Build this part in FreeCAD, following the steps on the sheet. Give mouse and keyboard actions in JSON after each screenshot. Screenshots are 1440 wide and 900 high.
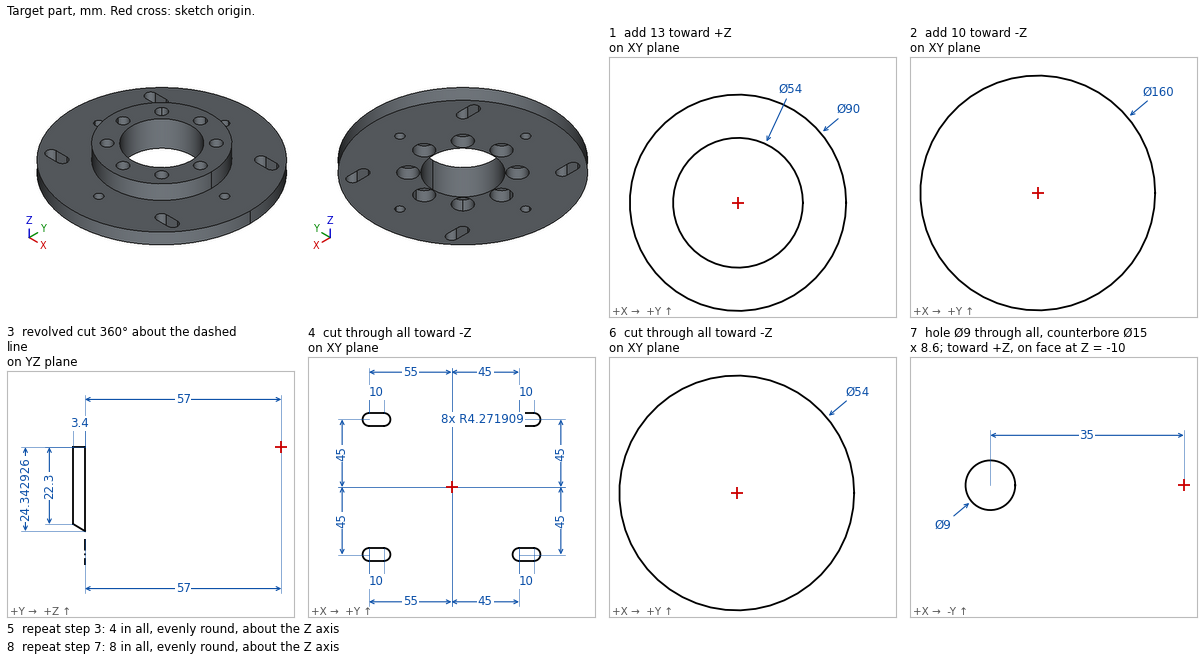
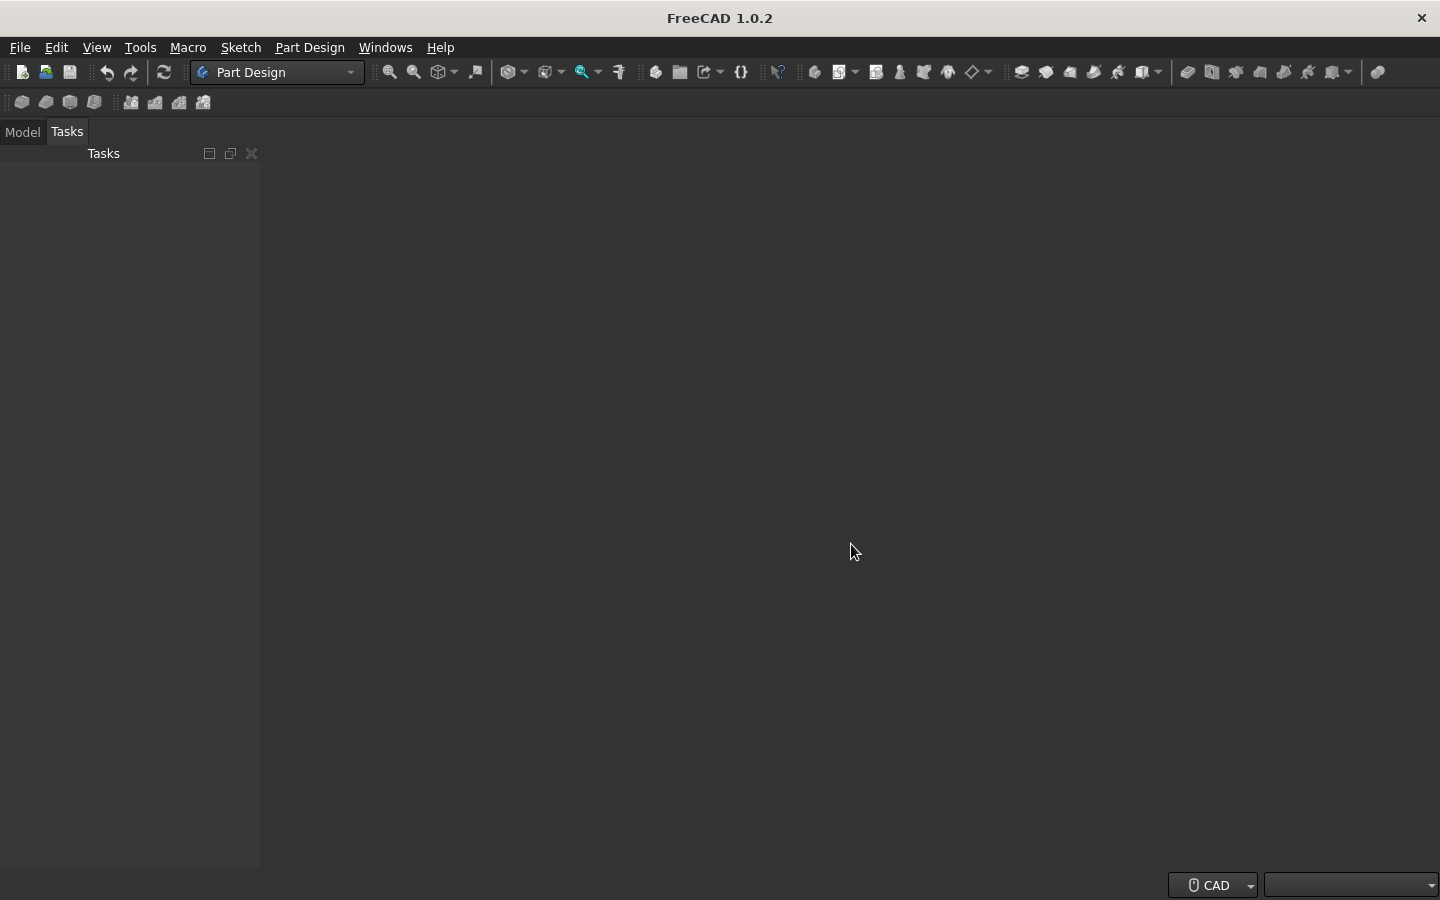
{"action": "key", "text": "ctrl+n"}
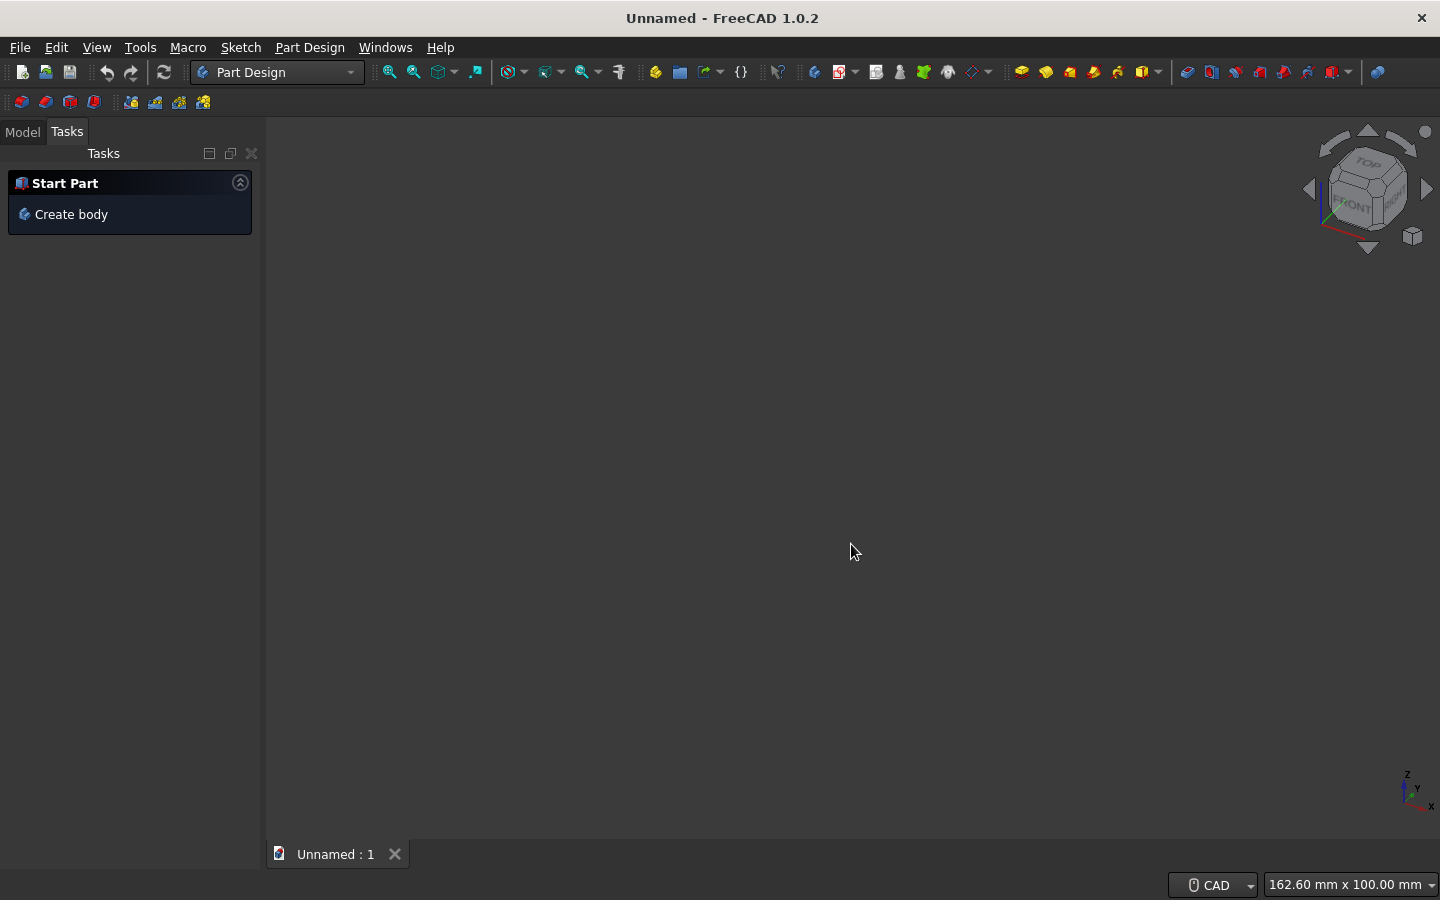
{"action": "left_click", "coordinate": [840, 72]}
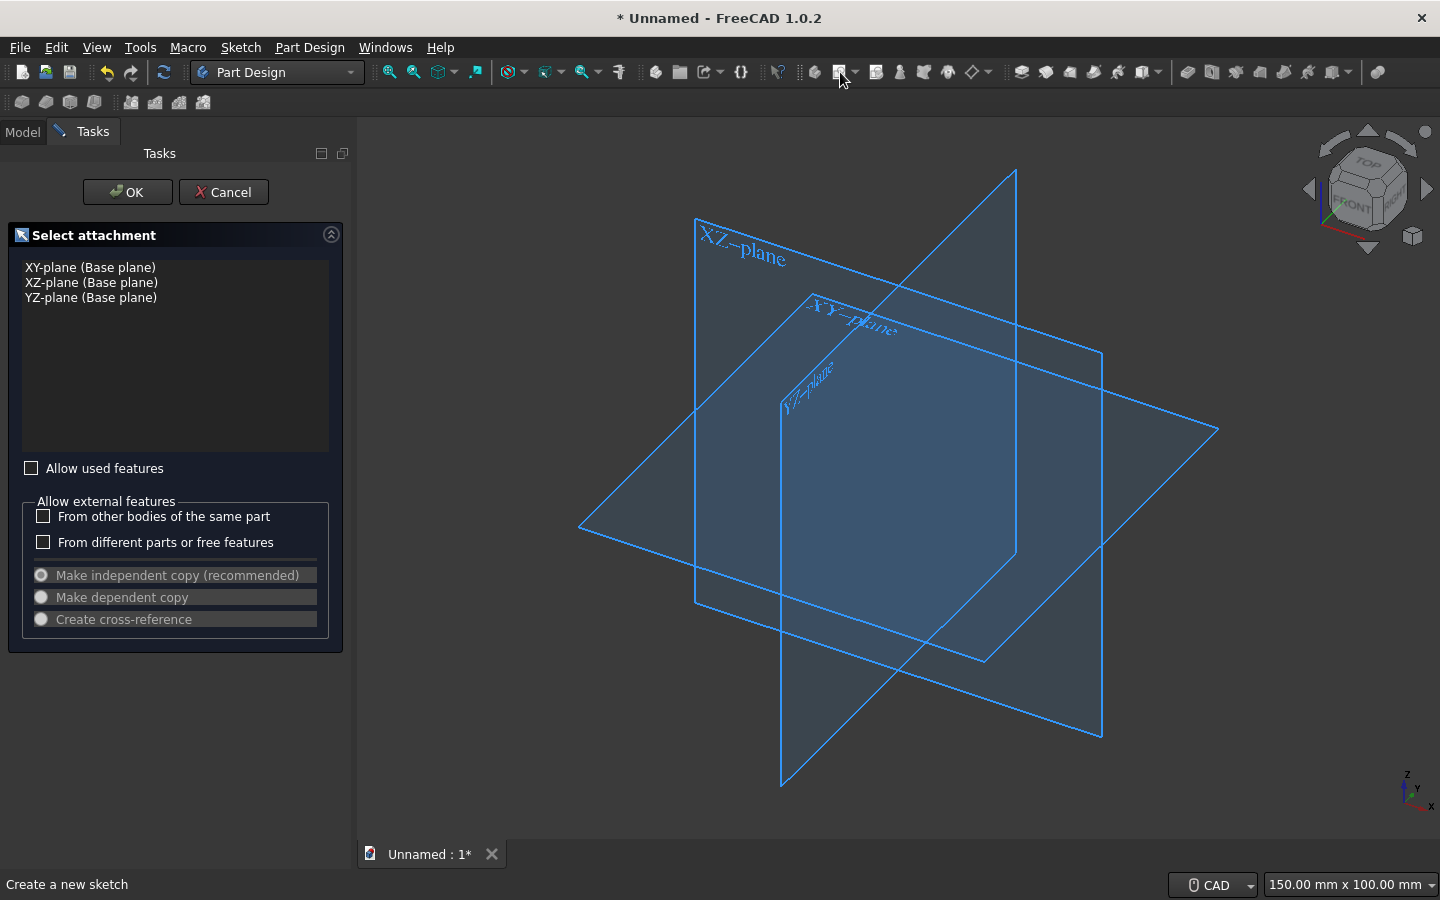
{"action": "left_click", "coordinate": [82, 268]}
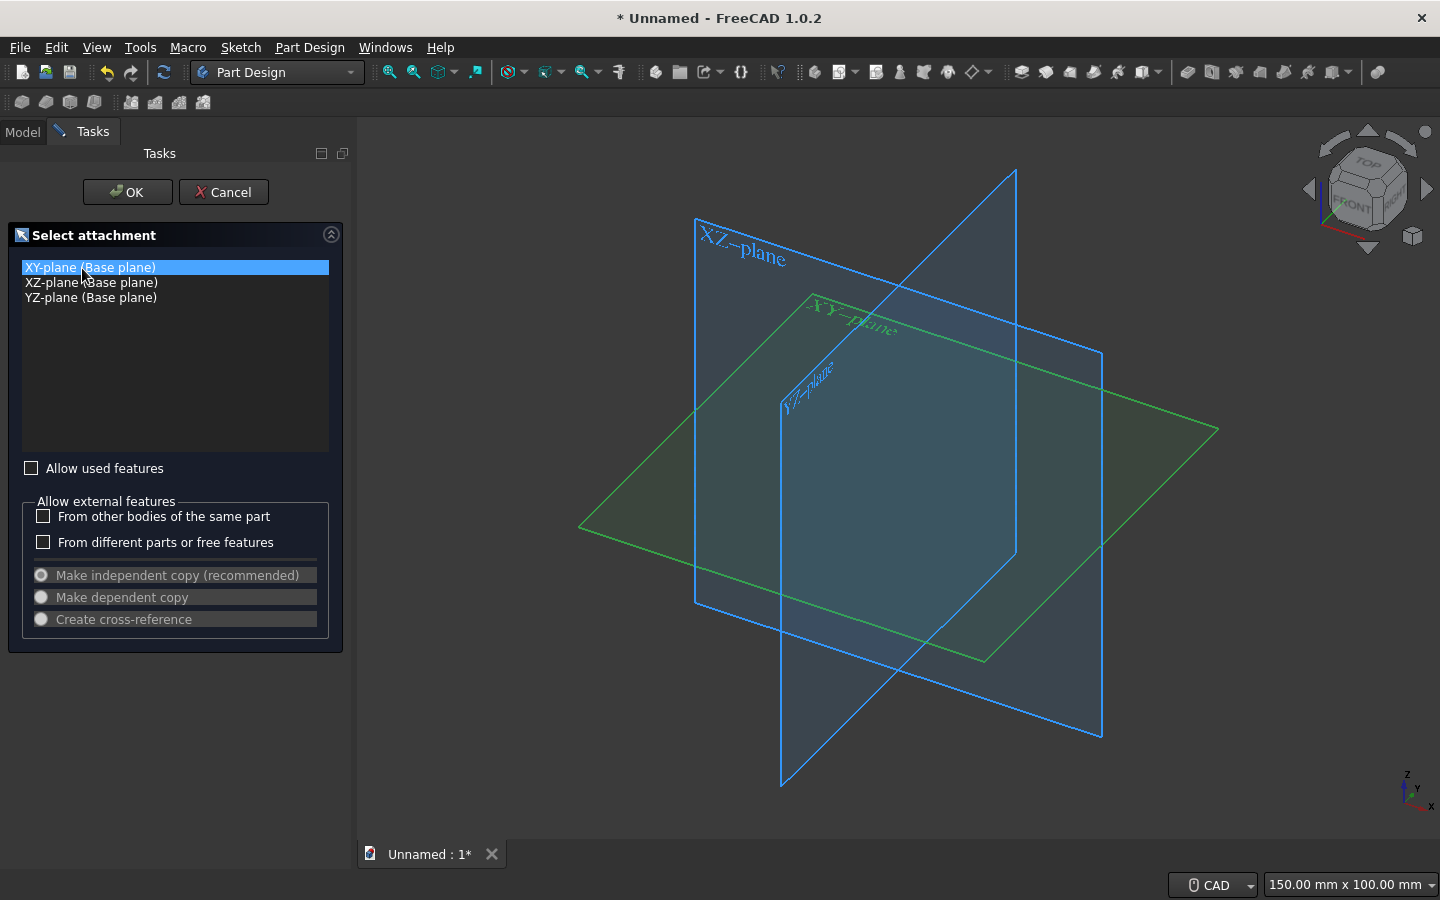
{"action": "left_click", "coordinate": [128, 192]}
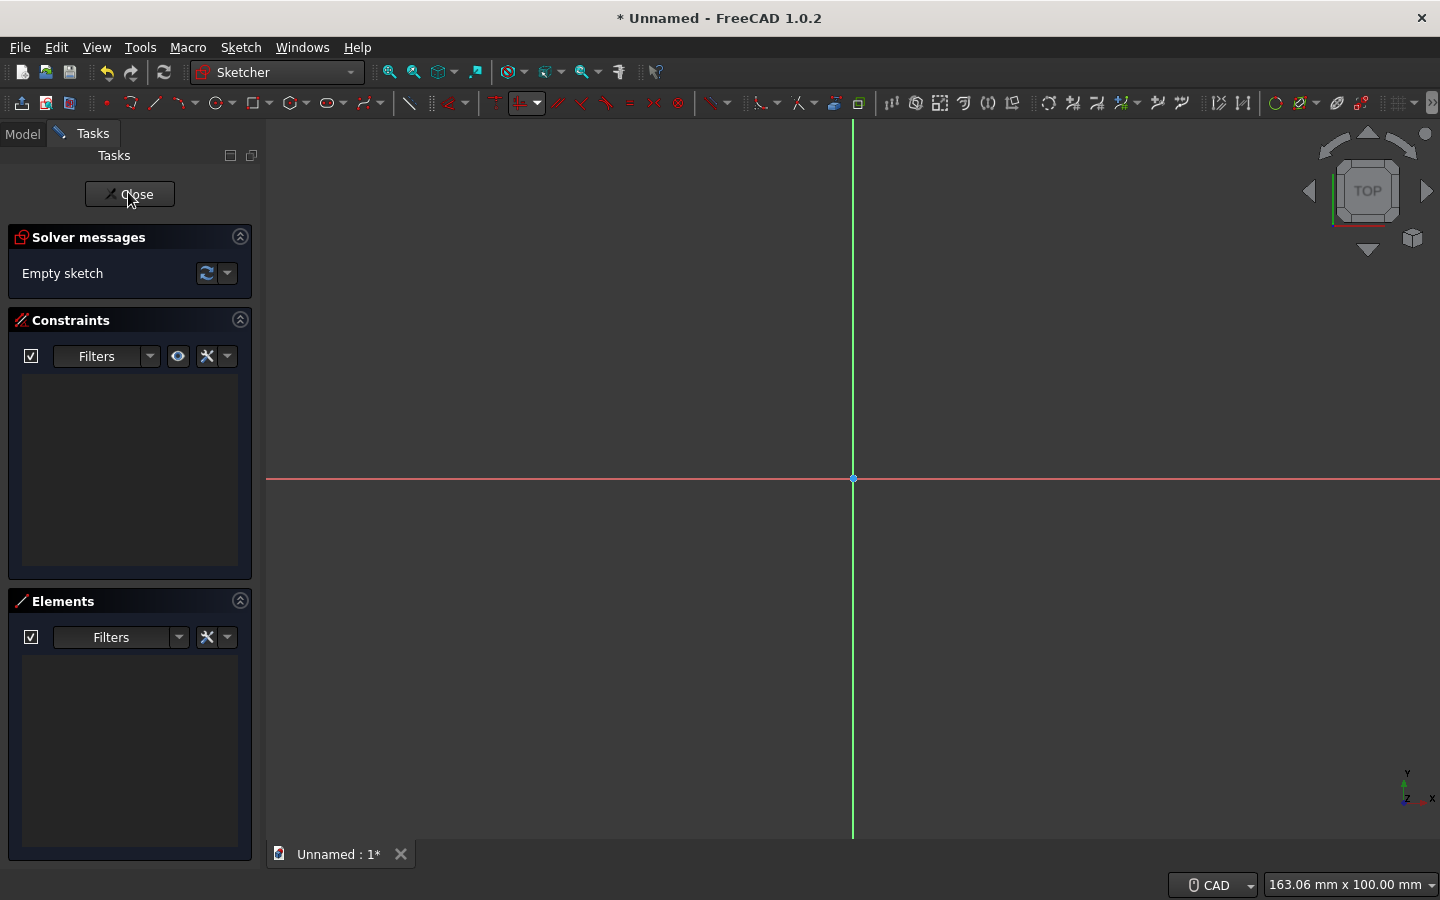
{"action": "scroll", "coordinate": [645, 479], "scroll_direction": "down", "scroll_amount": 2}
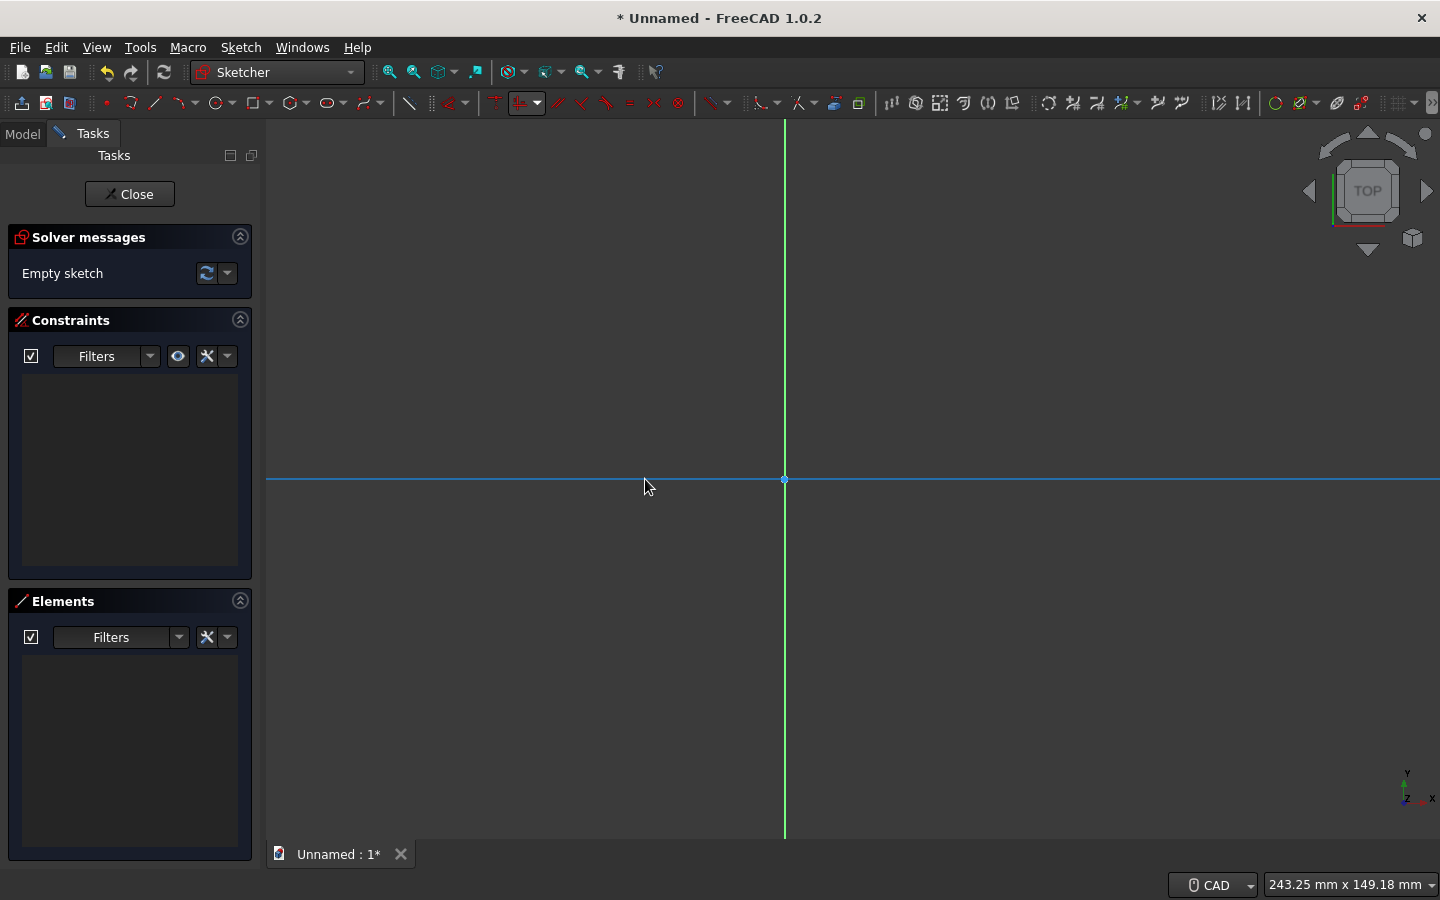
{"action": "left_click", "coordinate": [216, 104]}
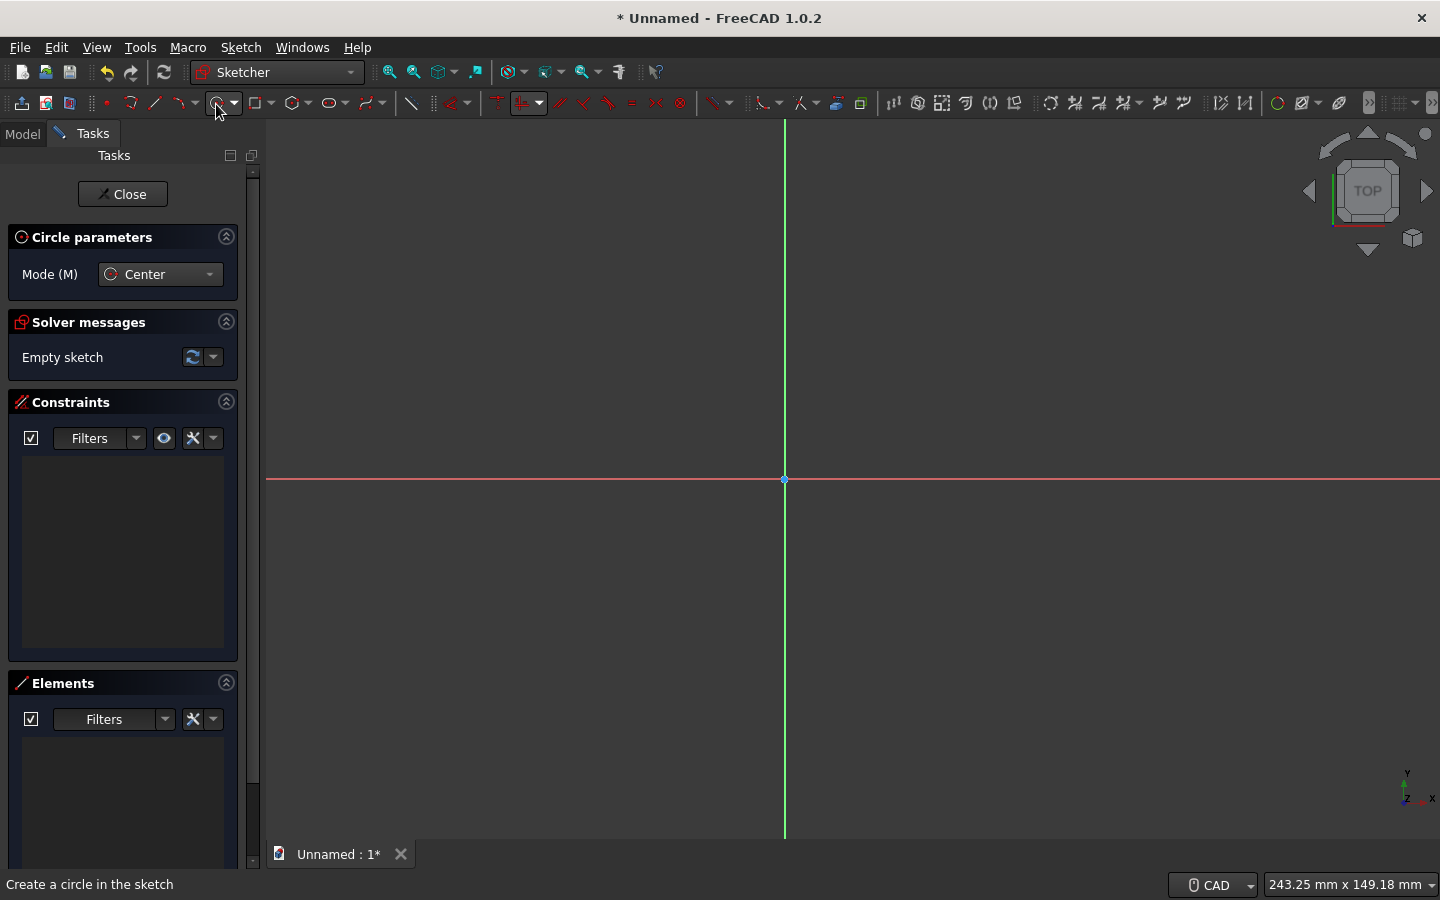
{"action": "left_click", "coordinate": [785, 479]}
{"action": "mouse_move", "coordinate": [938, 326]}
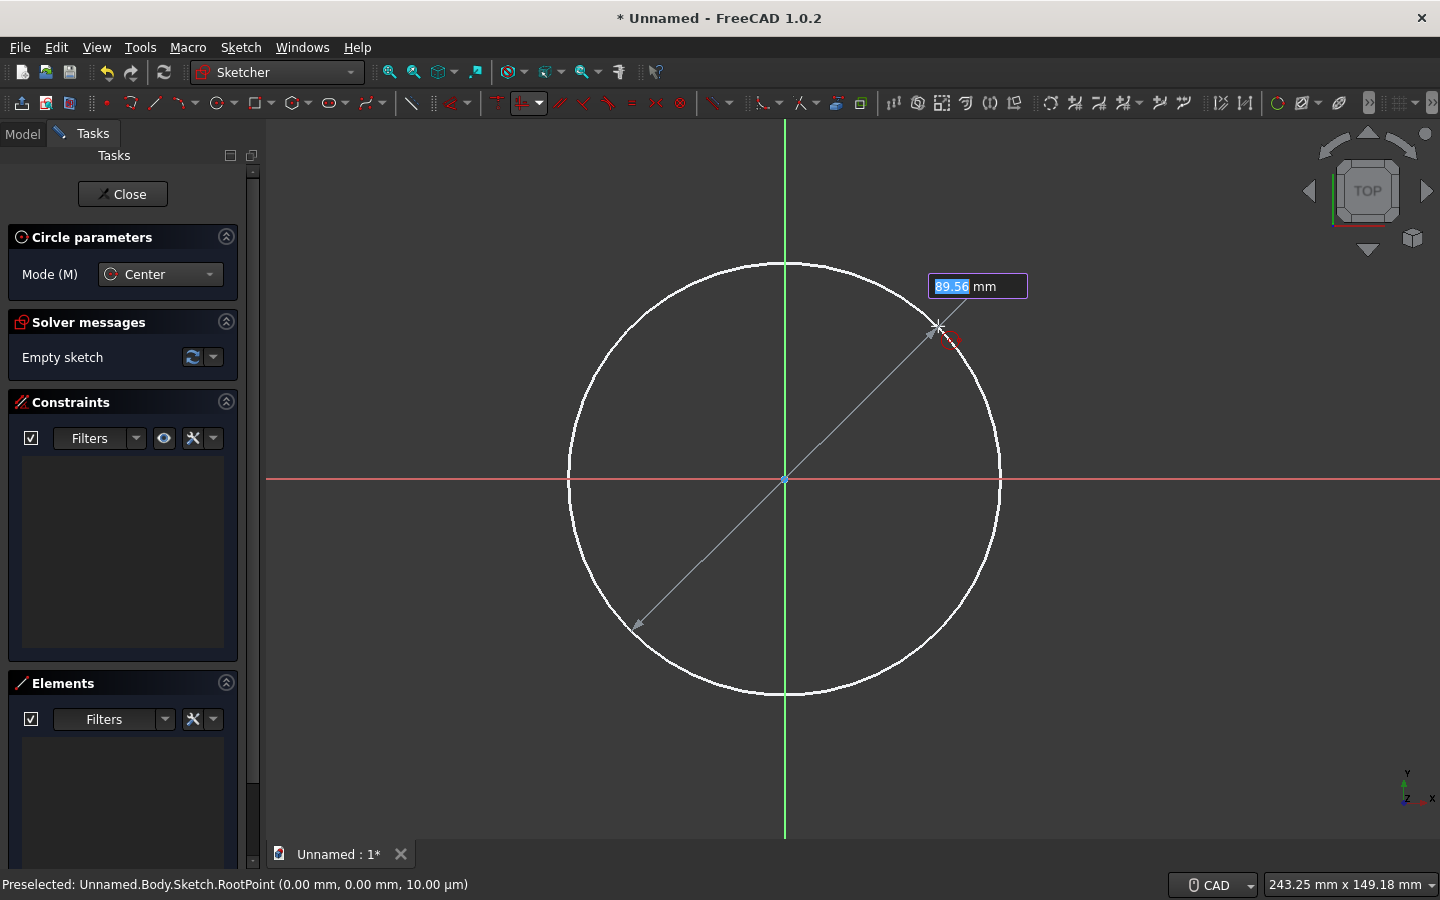
{"action": "type", "text": "90"}
{"action": "key", "text": "Return"}